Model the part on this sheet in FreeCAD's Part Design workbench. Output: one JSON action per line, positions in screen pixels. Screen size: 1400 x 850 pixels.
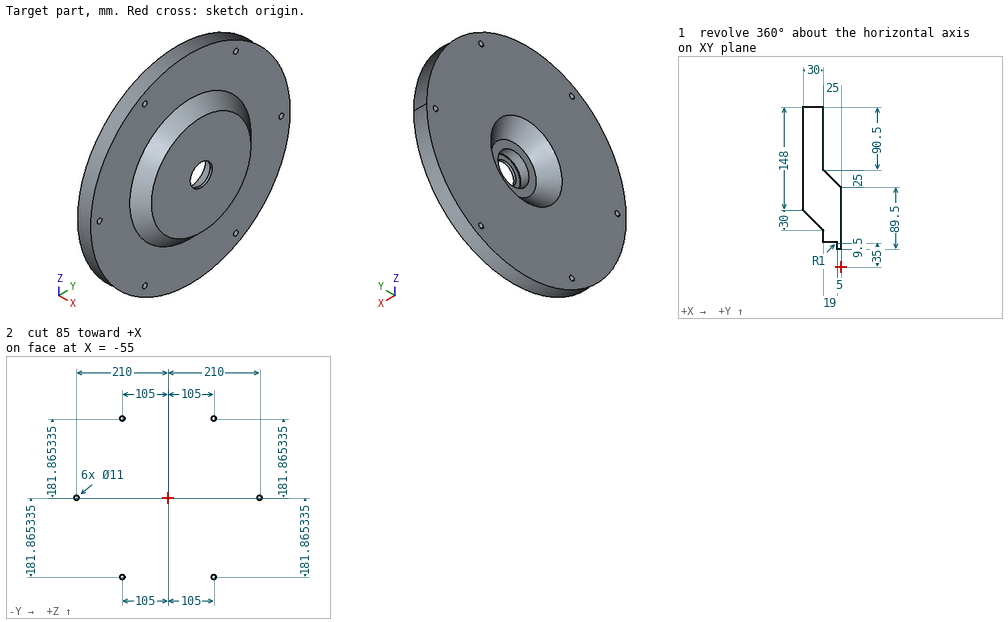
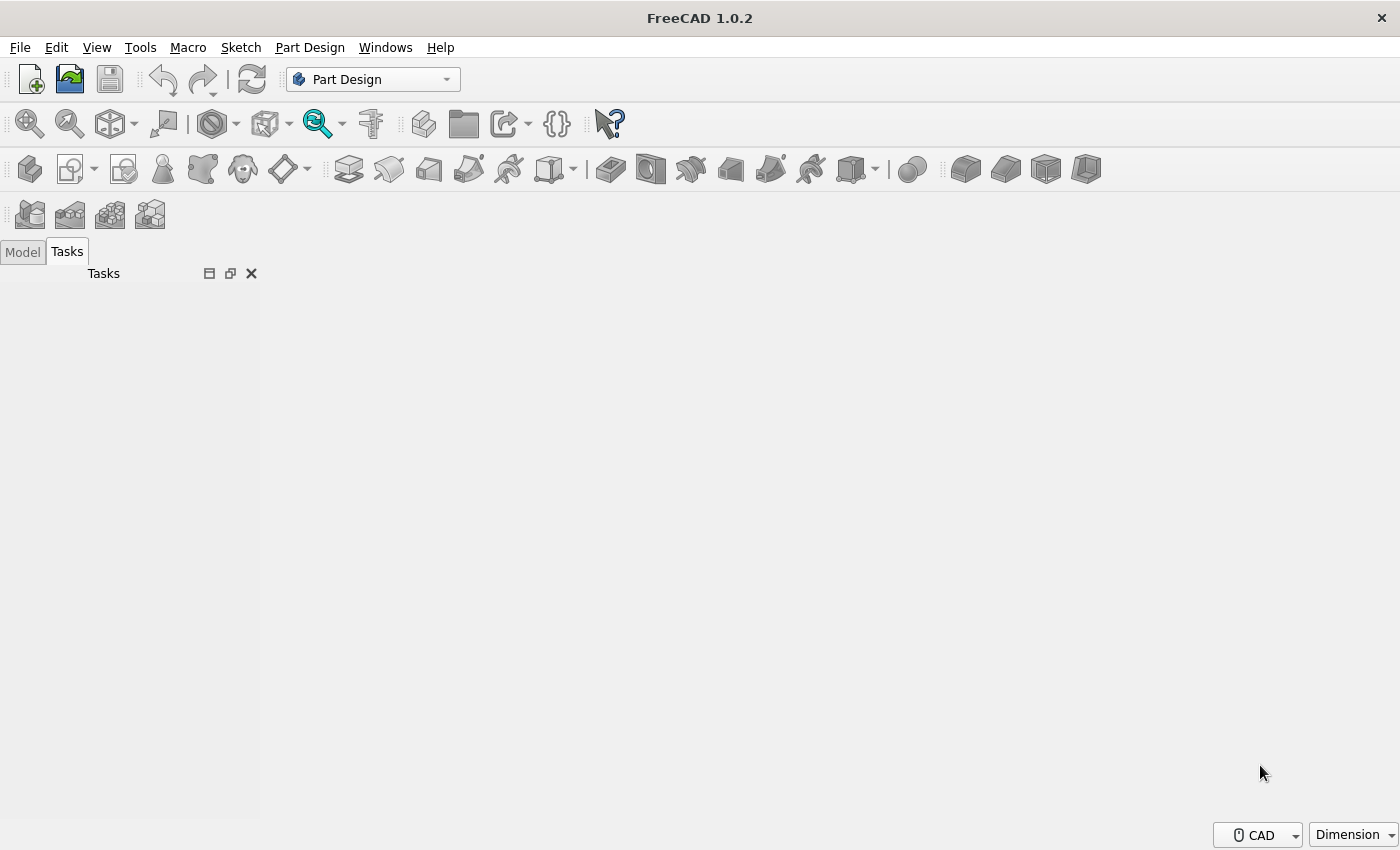
{"action": "left_click", "coordinate": [216, 80]}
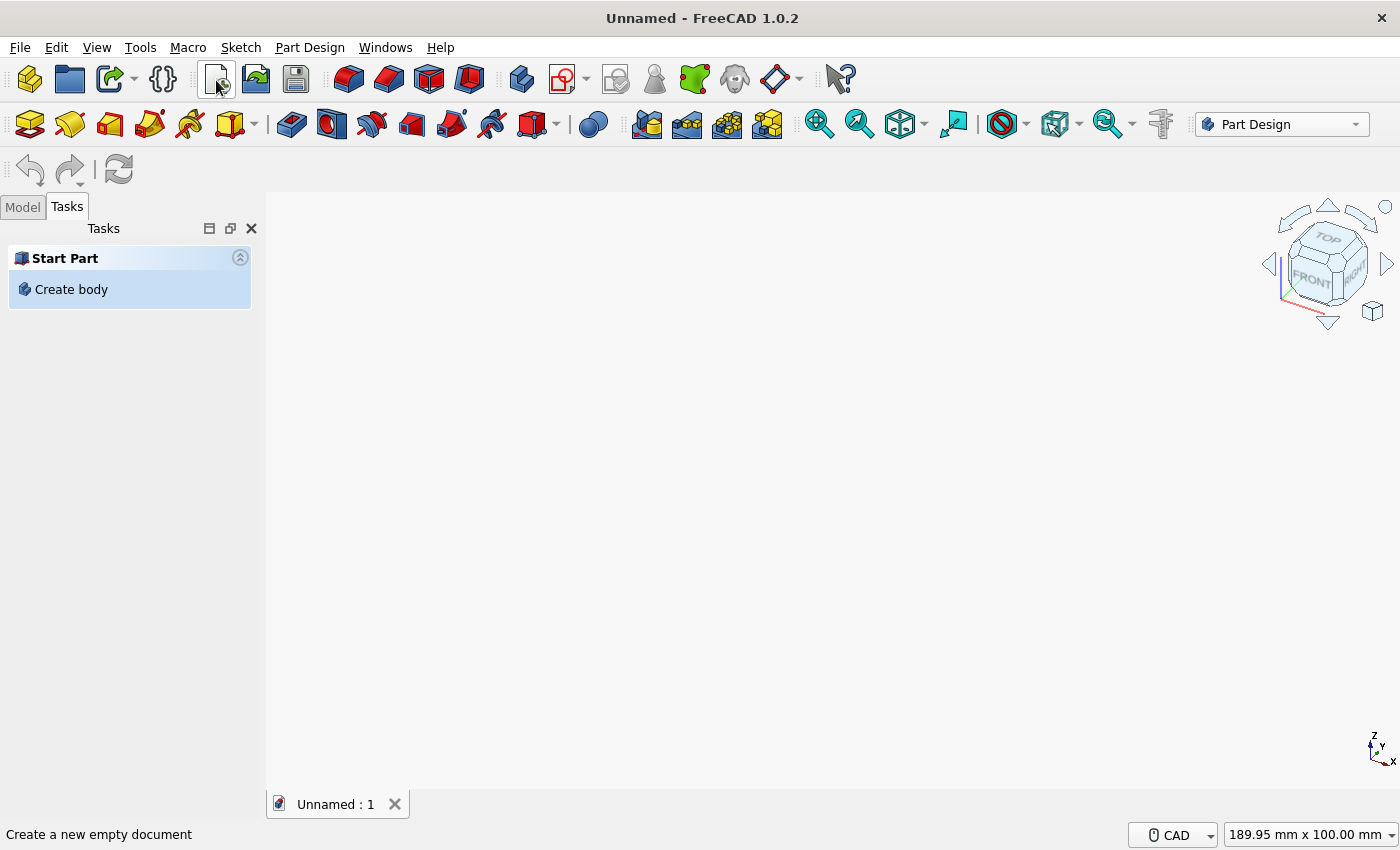
{"action": "left_click", "coordinate": [562, 80]}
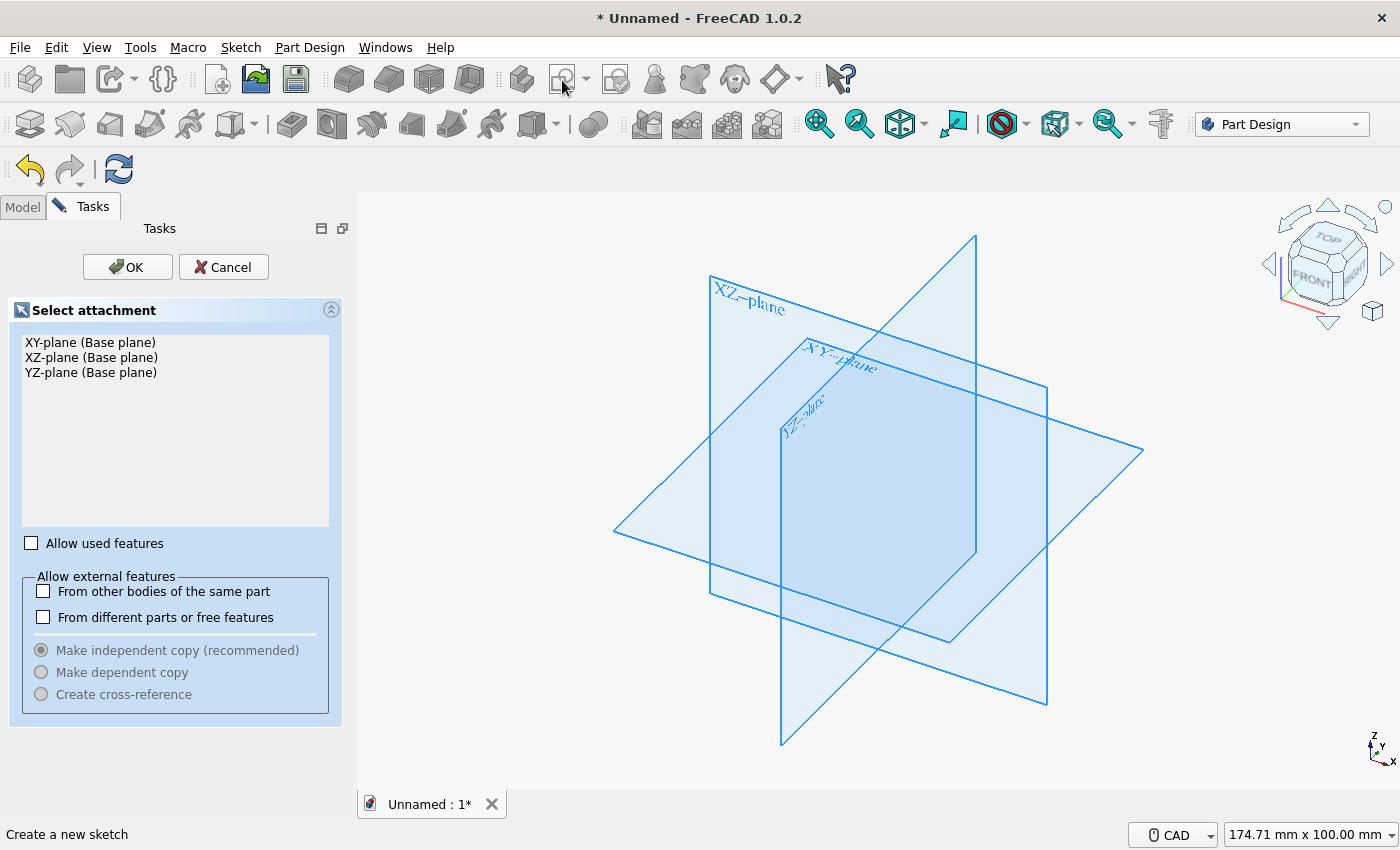
{"action": "left_click", "coordinate": [82, 342]}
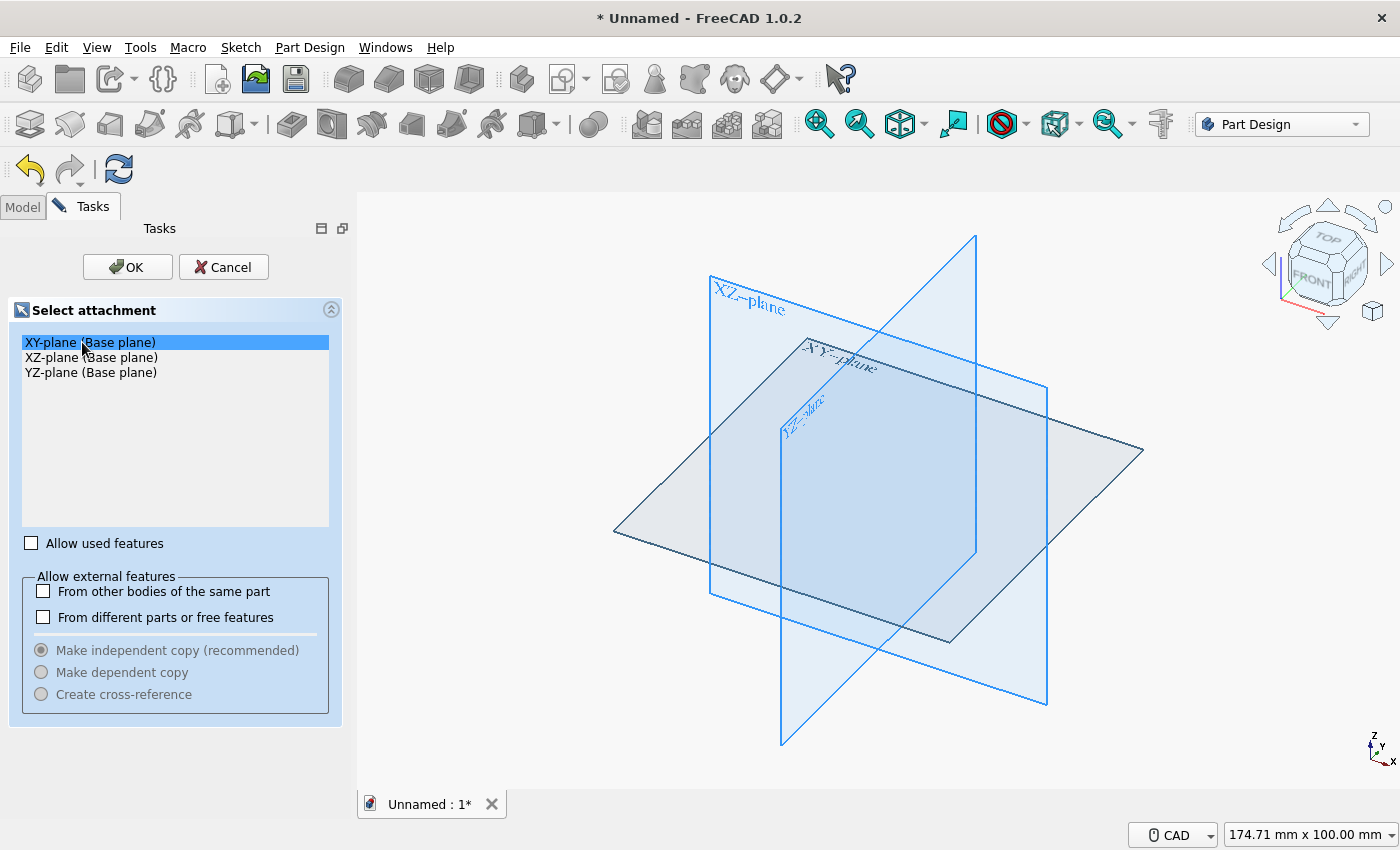
{"action": "left_click", "coordinate": [128, 267]}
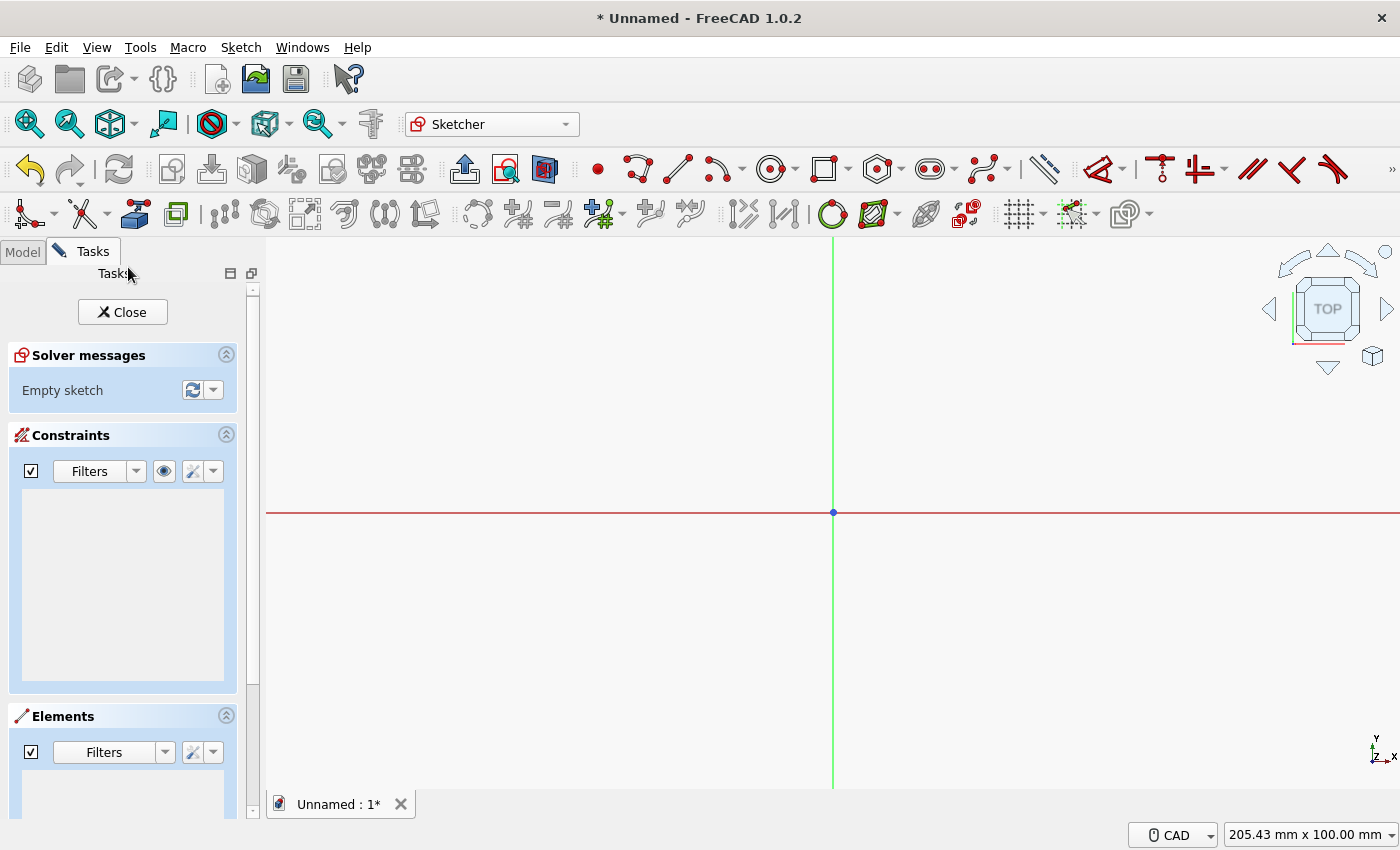
{"action": "scroll", "coordinate": [800, 761], "scroll_direction": "down", "scroll_amount": 6}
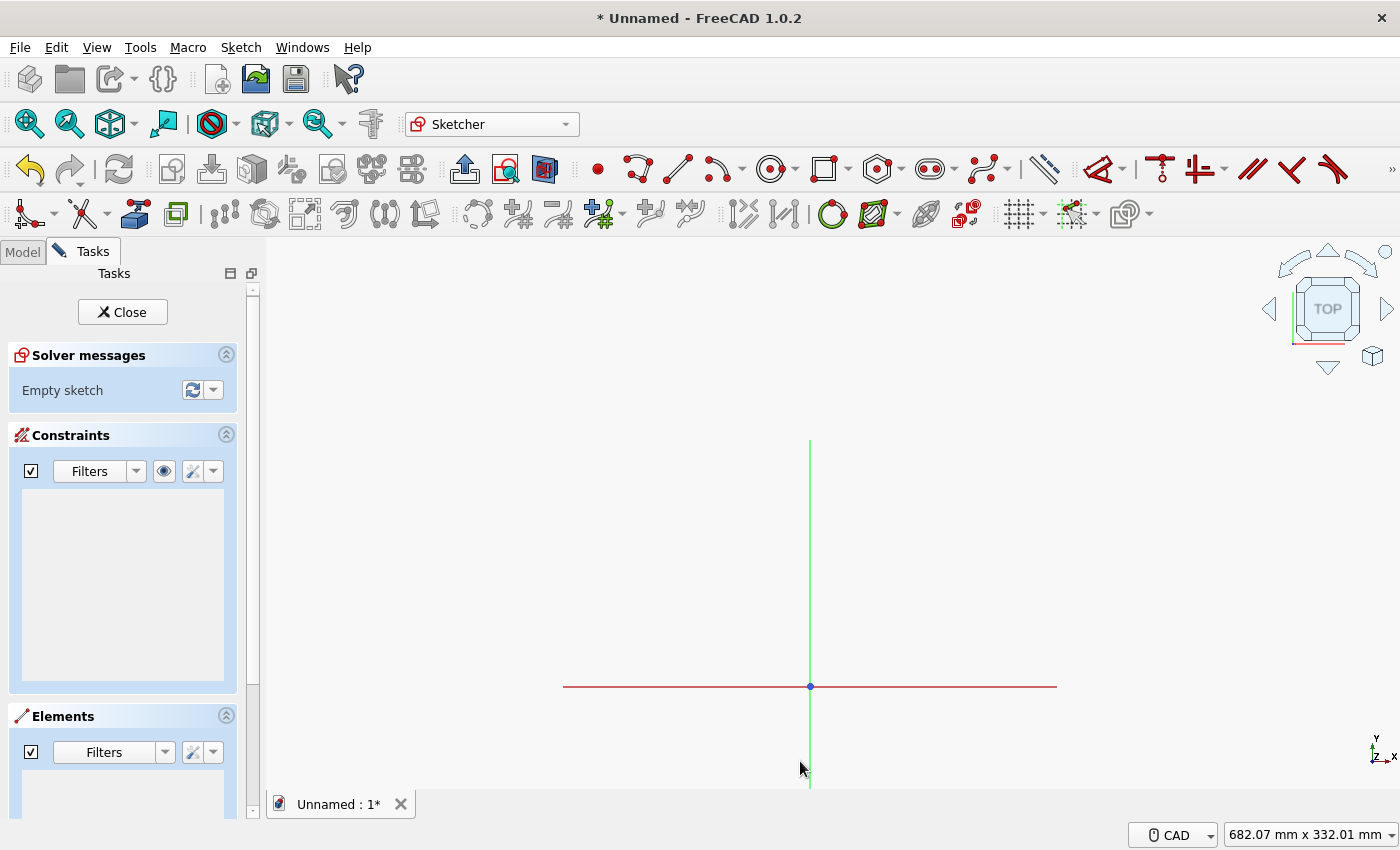
{"action": "left_click", "coordinate": [638, 170]}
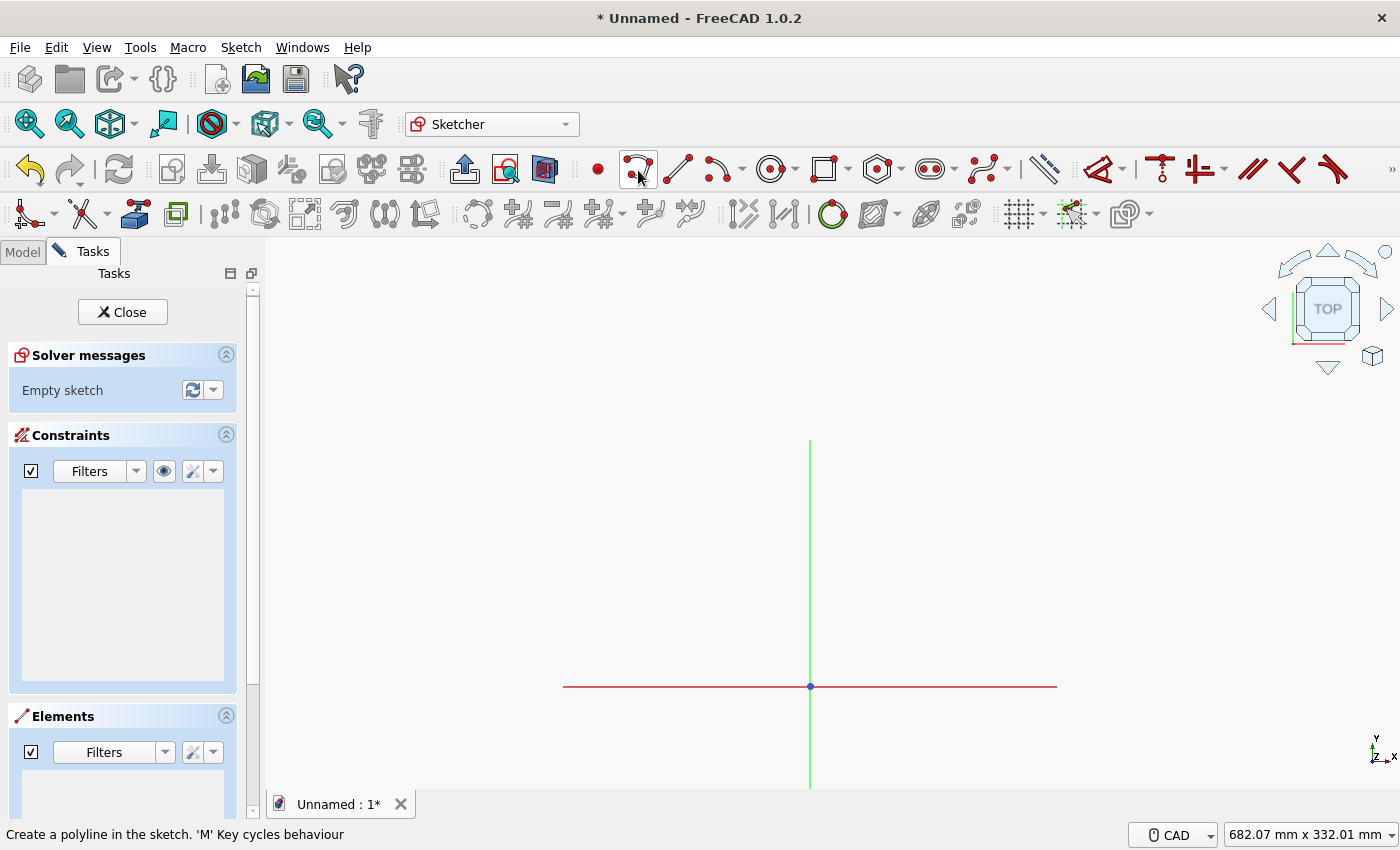
{"action": "scroll", "coordinate": [802, 629], "scroll_direction": "up", "scroll_amount": 4}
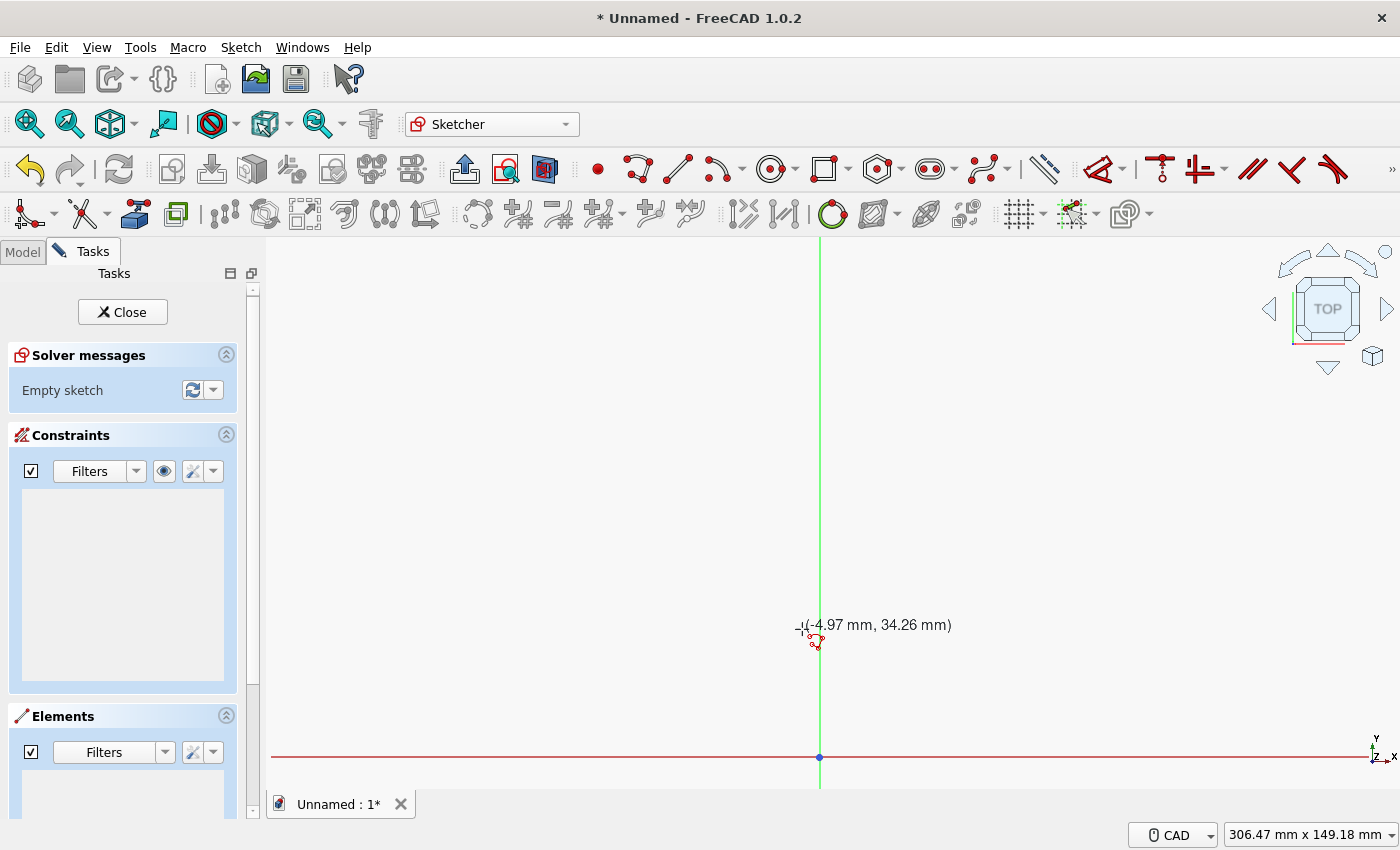
{"action": "left_click", "coordinate": [801, 628]}
{"action": "left_click", "coordinate": [801, 663]}
{"action": "left_click", "coordinate": [820, 663]}
{"action": "left_click", "coordinate": [811, 332]}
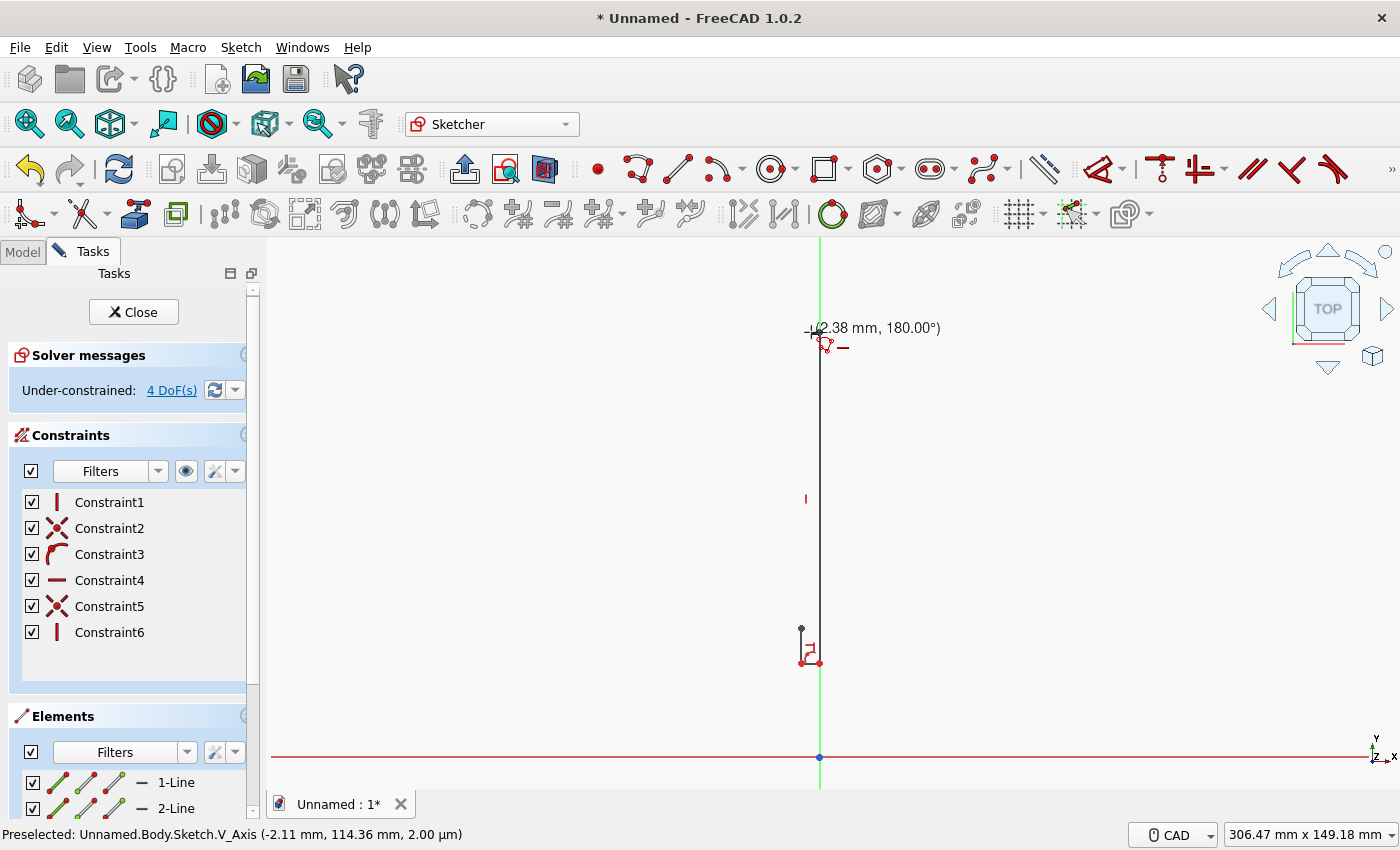
{"action": "scroll", "coordinate": [802, 662], "scroll_direction": "down", "scroll_amount": 4}